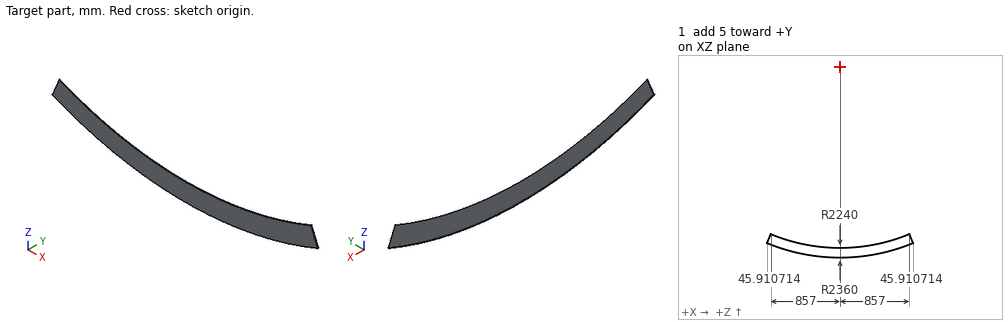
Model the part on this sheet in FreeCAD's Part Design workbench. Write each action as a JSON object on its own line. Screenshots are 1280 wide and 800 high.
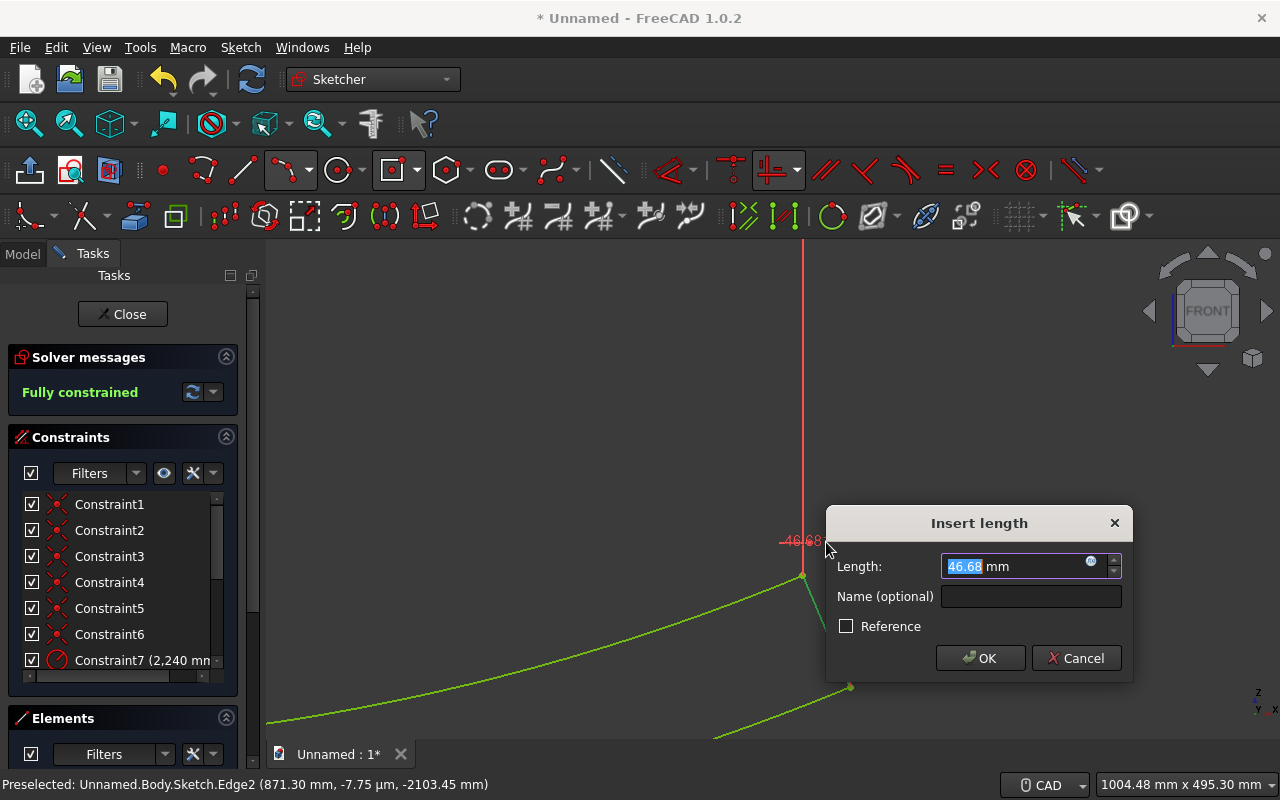
{"action": "type", "text": "45.910714"}
{"action": "key", "text": "Return"}
{"action": "key", "text": "Escape"}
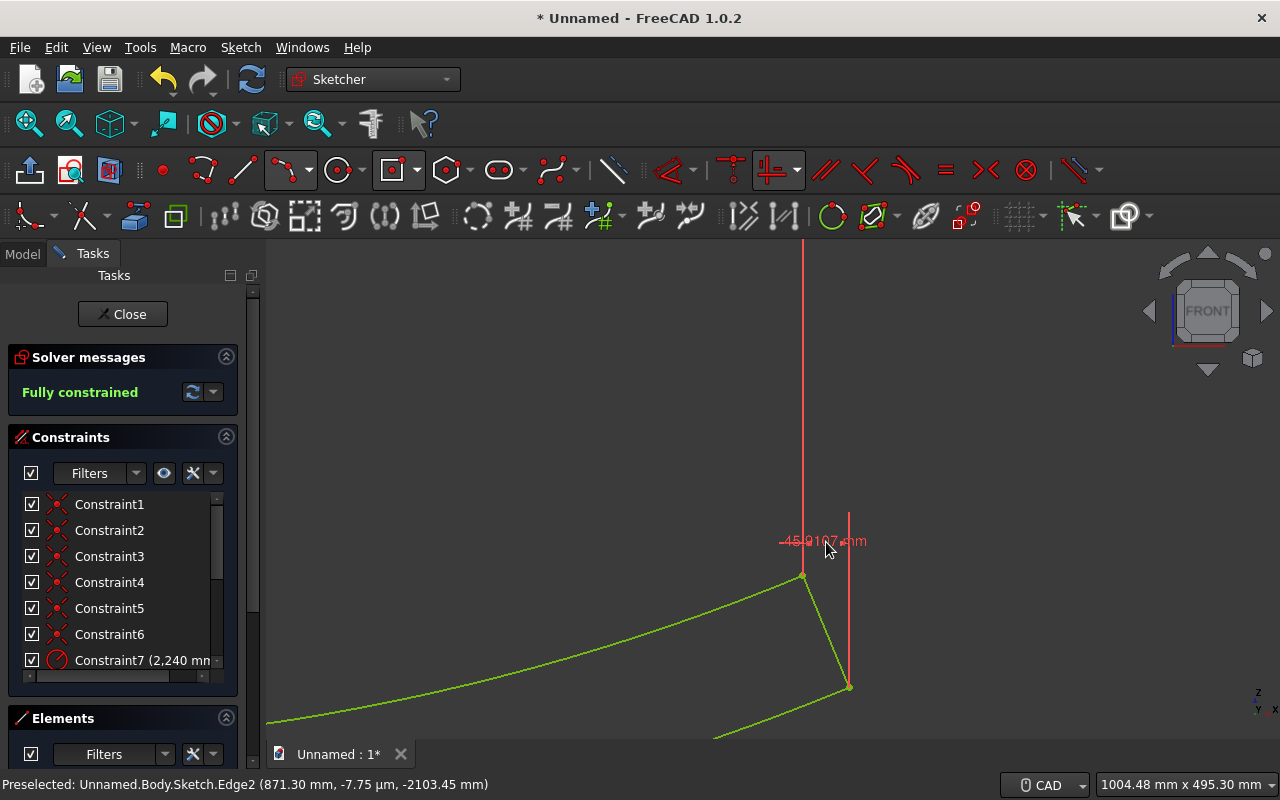
{"action": "left_click", "coordinate": [123, 314]}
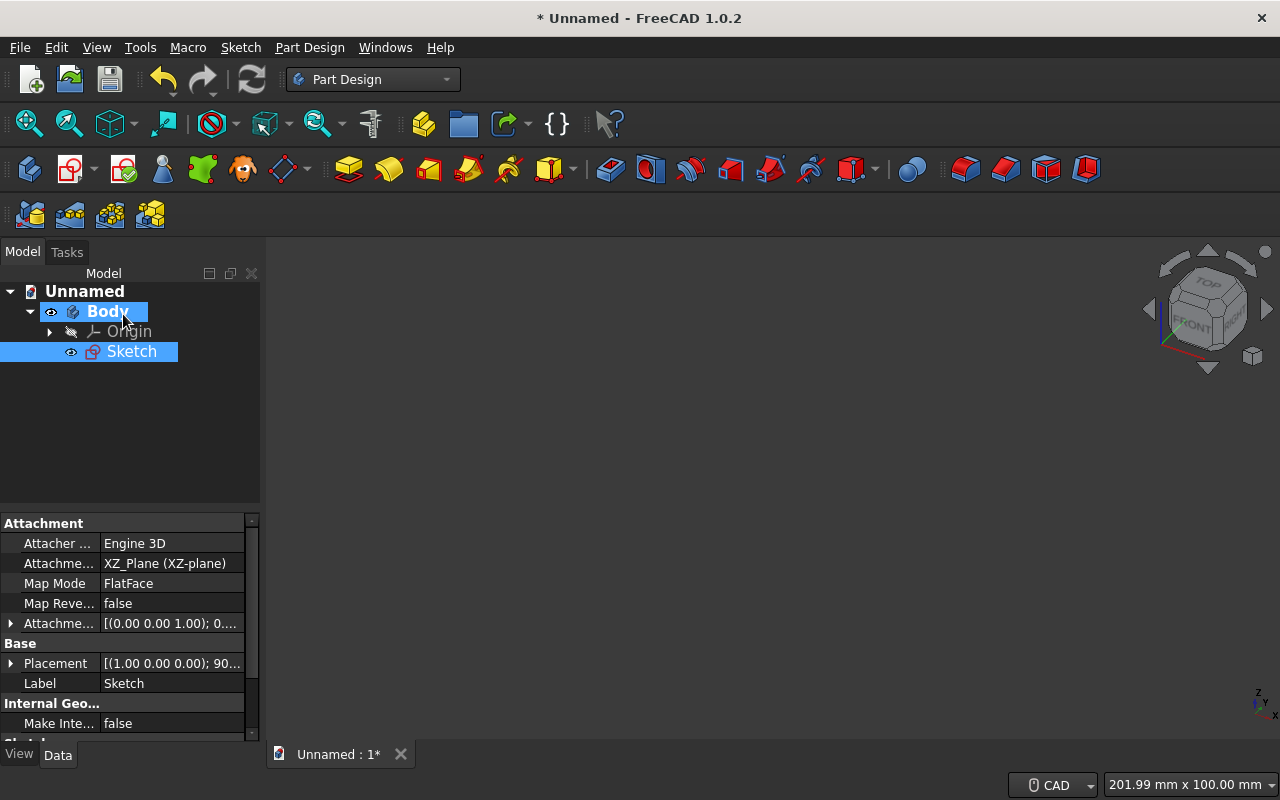
{"action": "left_click", "coordinate": [350, 170]}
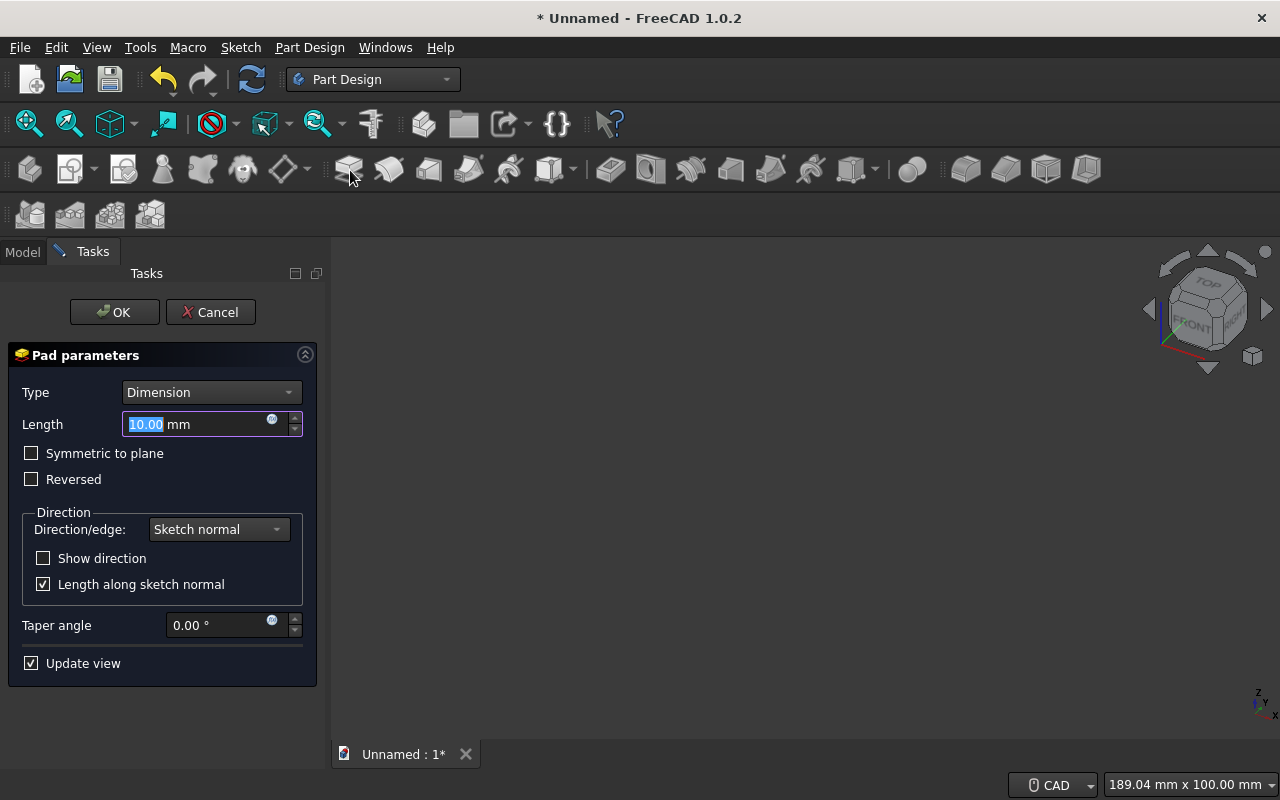
{"action": "type", "text": "5"}
{"action": "key", "text": "Tab"}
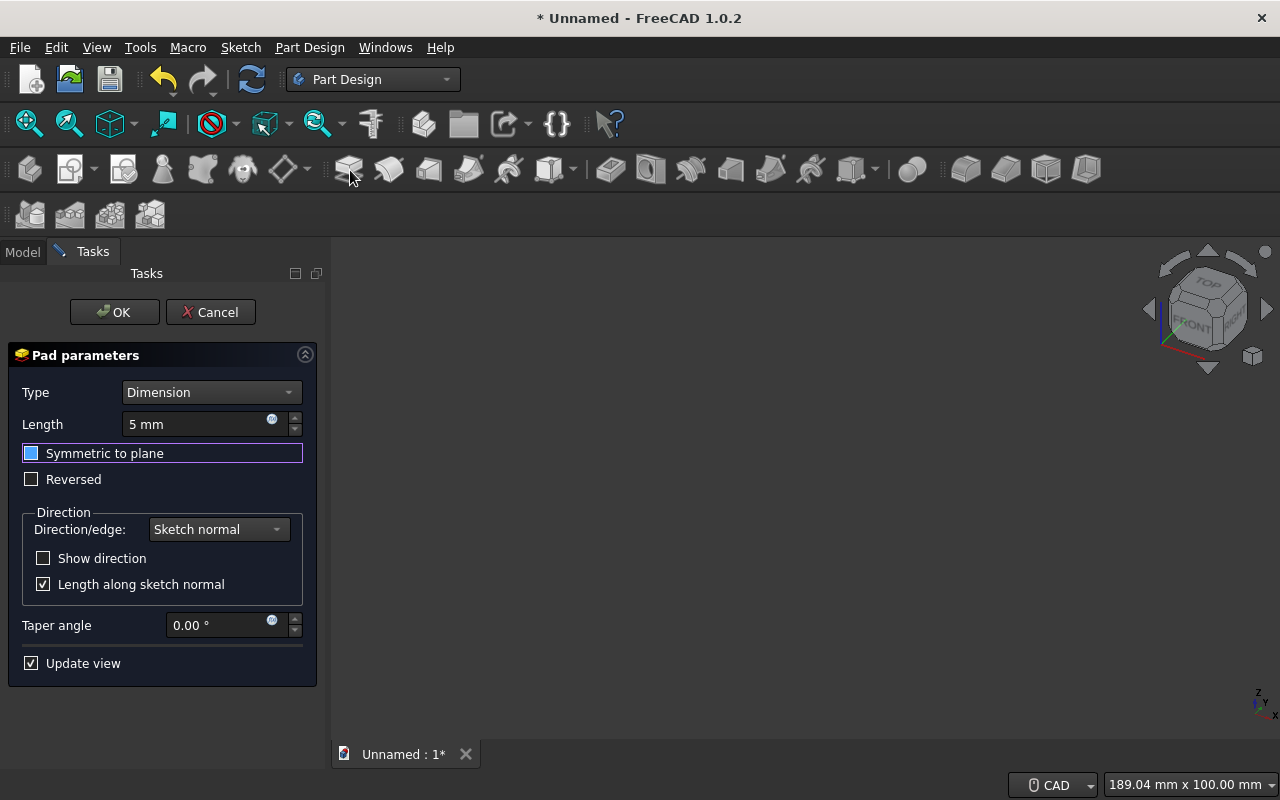
{"action": "left_click", "coordinate": [30, 479]}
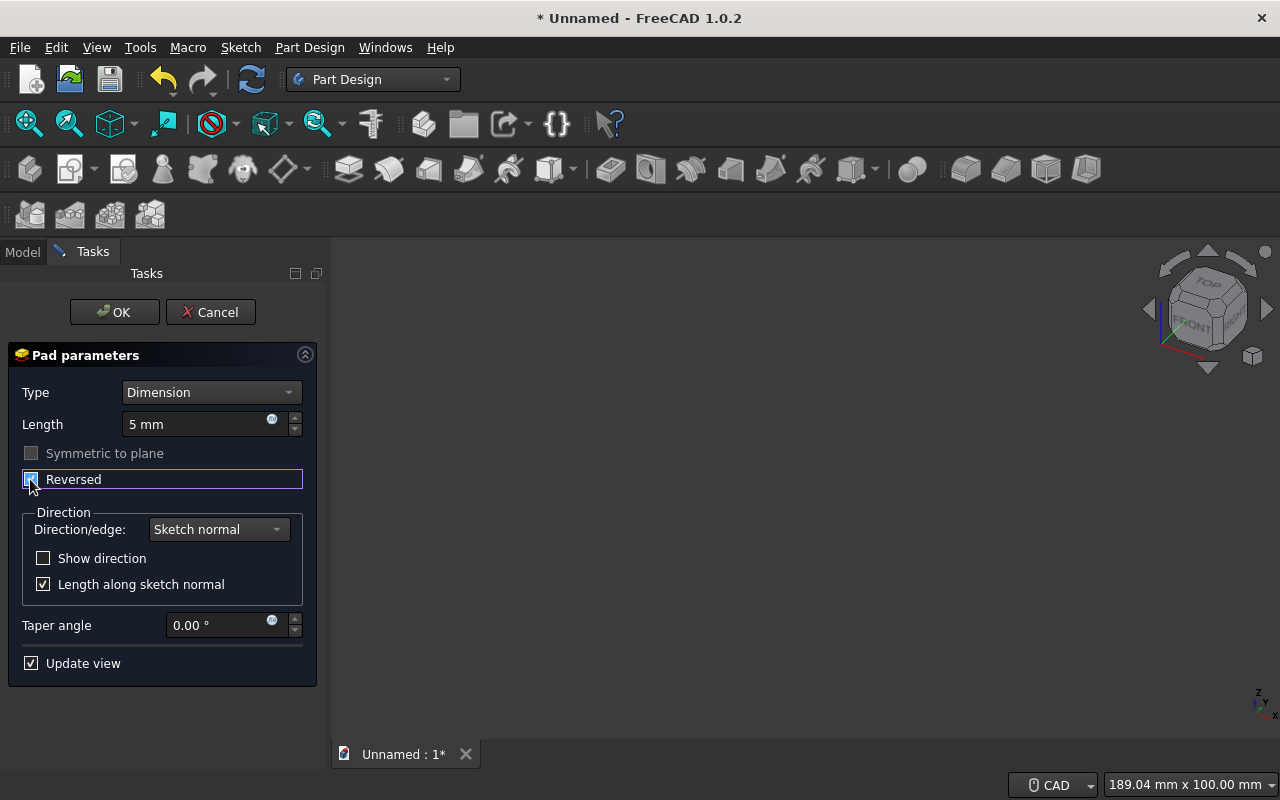
{"action": "left_click", "coordinate": [115, 312]}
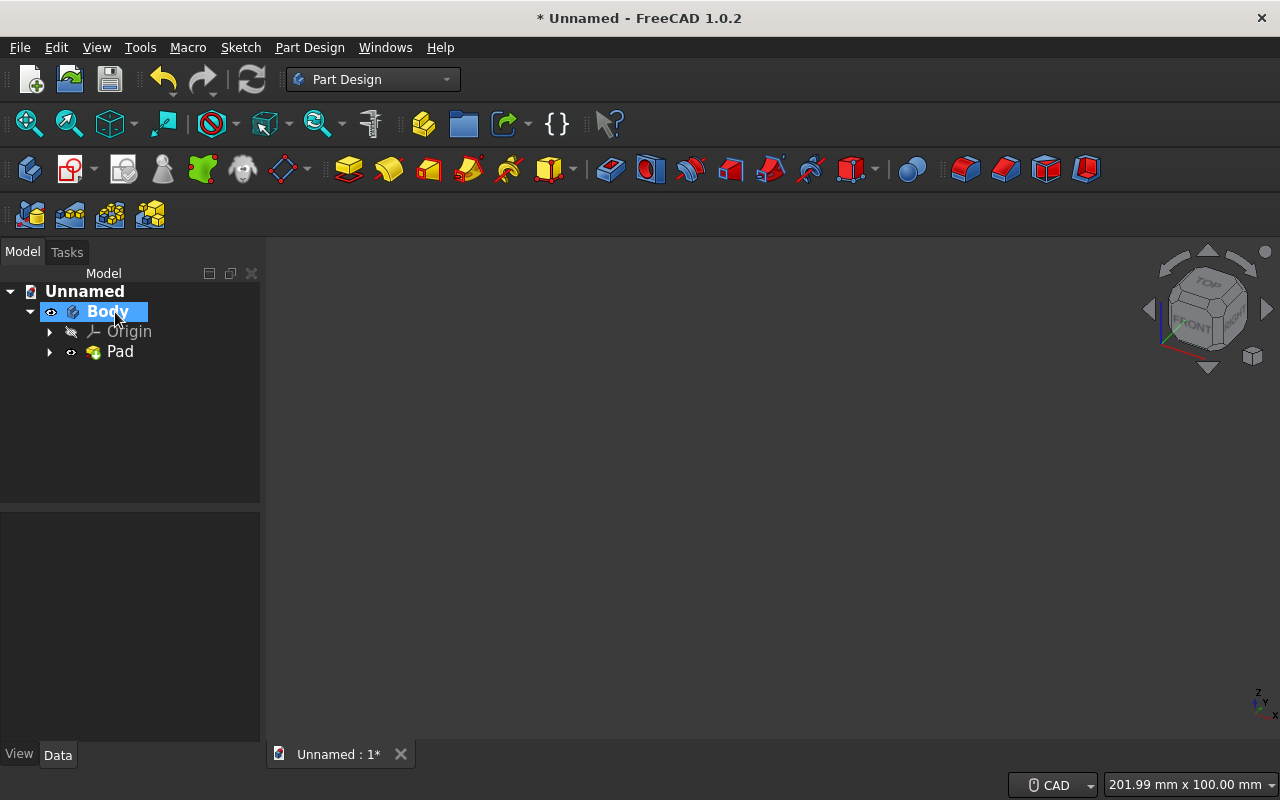
{"action": "key", "text": "0"}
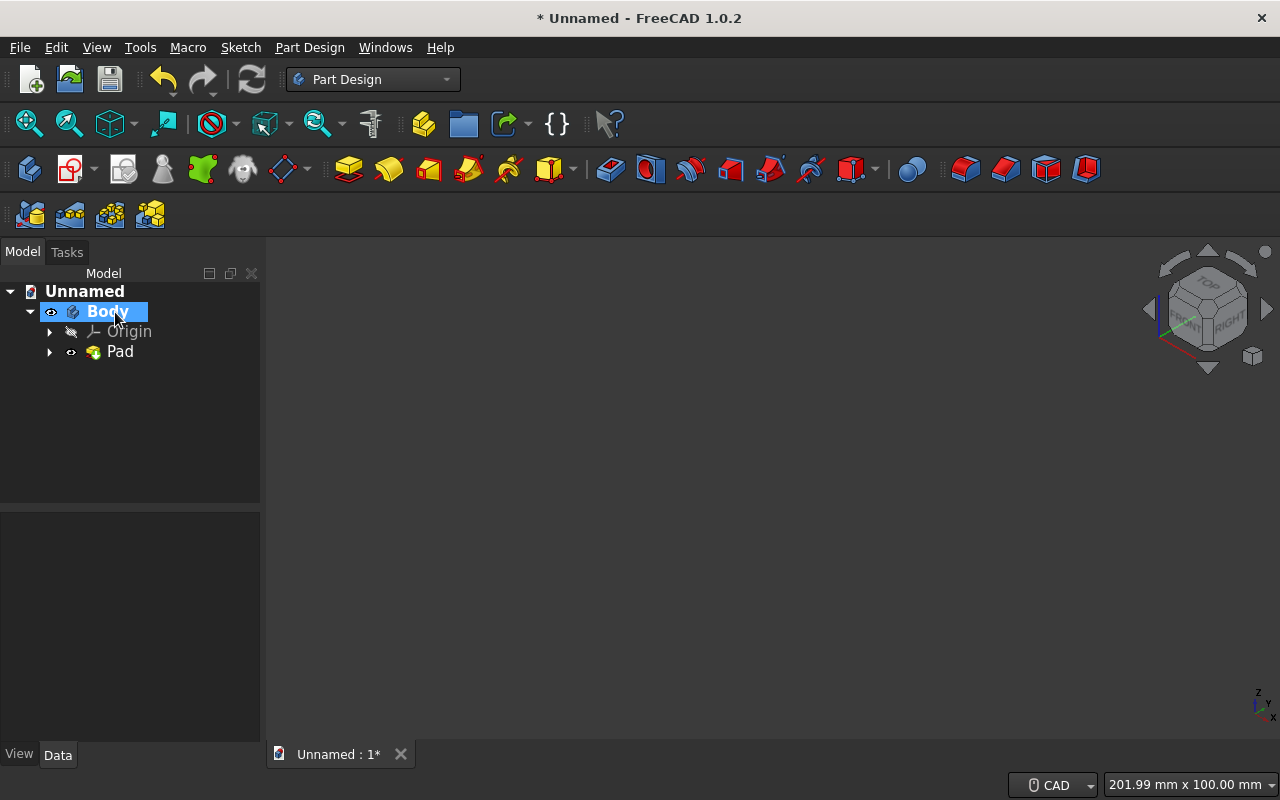
{"action": "left_click", "coordinate": [30, 124]}